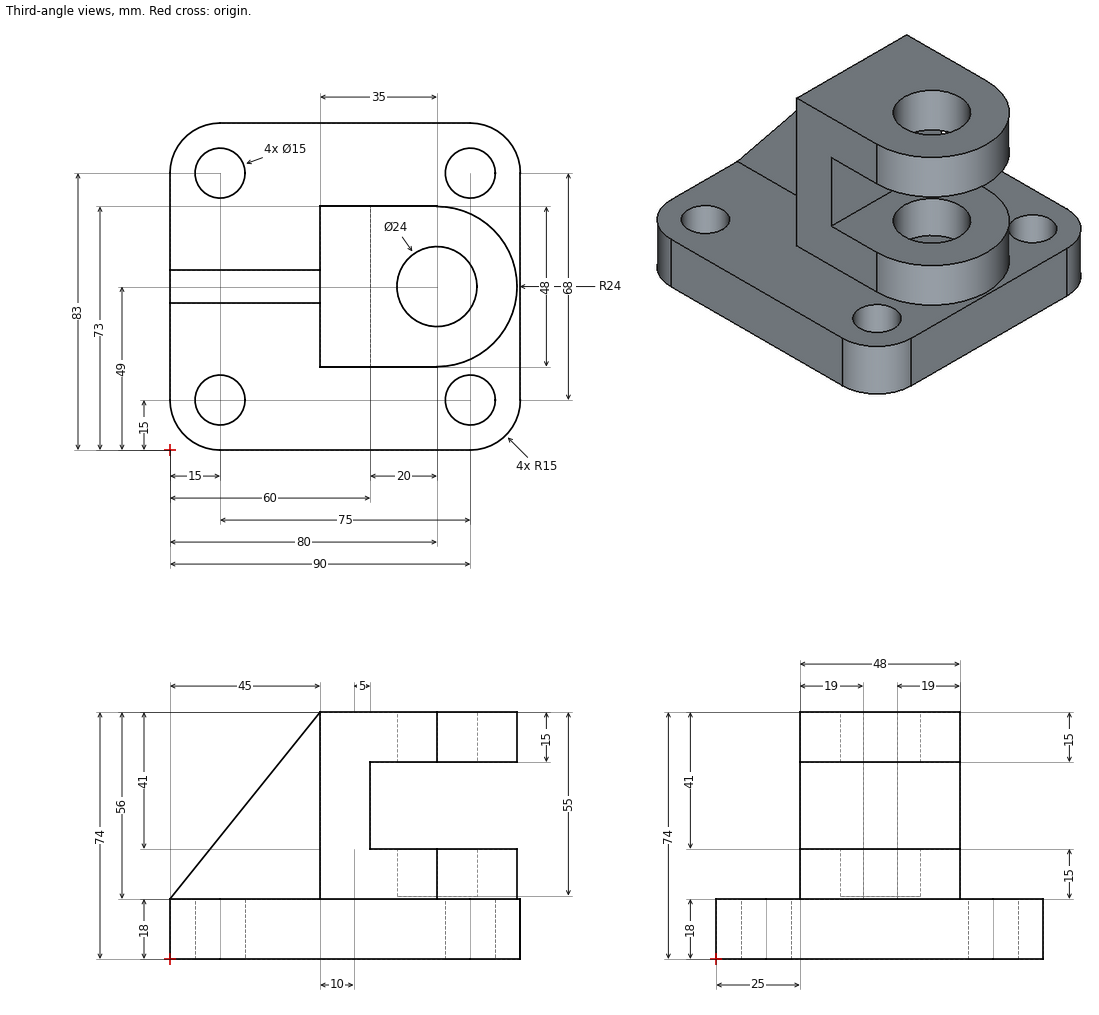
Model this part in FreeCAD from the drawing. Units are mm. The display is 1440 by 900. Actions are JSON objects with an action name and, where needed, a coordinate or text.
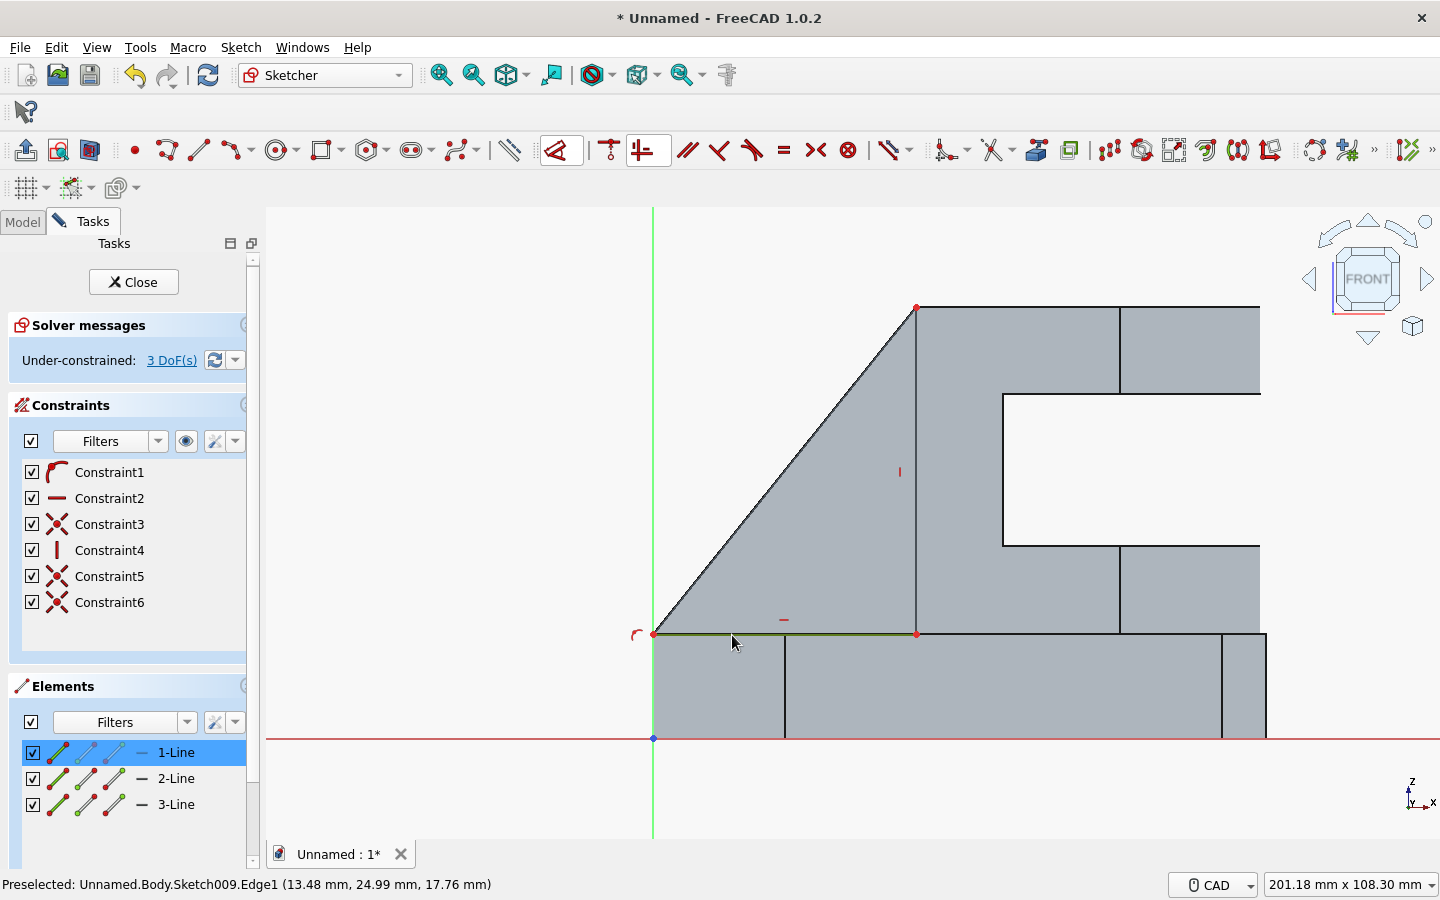
{"action": "left_click", "coordinate": [578, 150]}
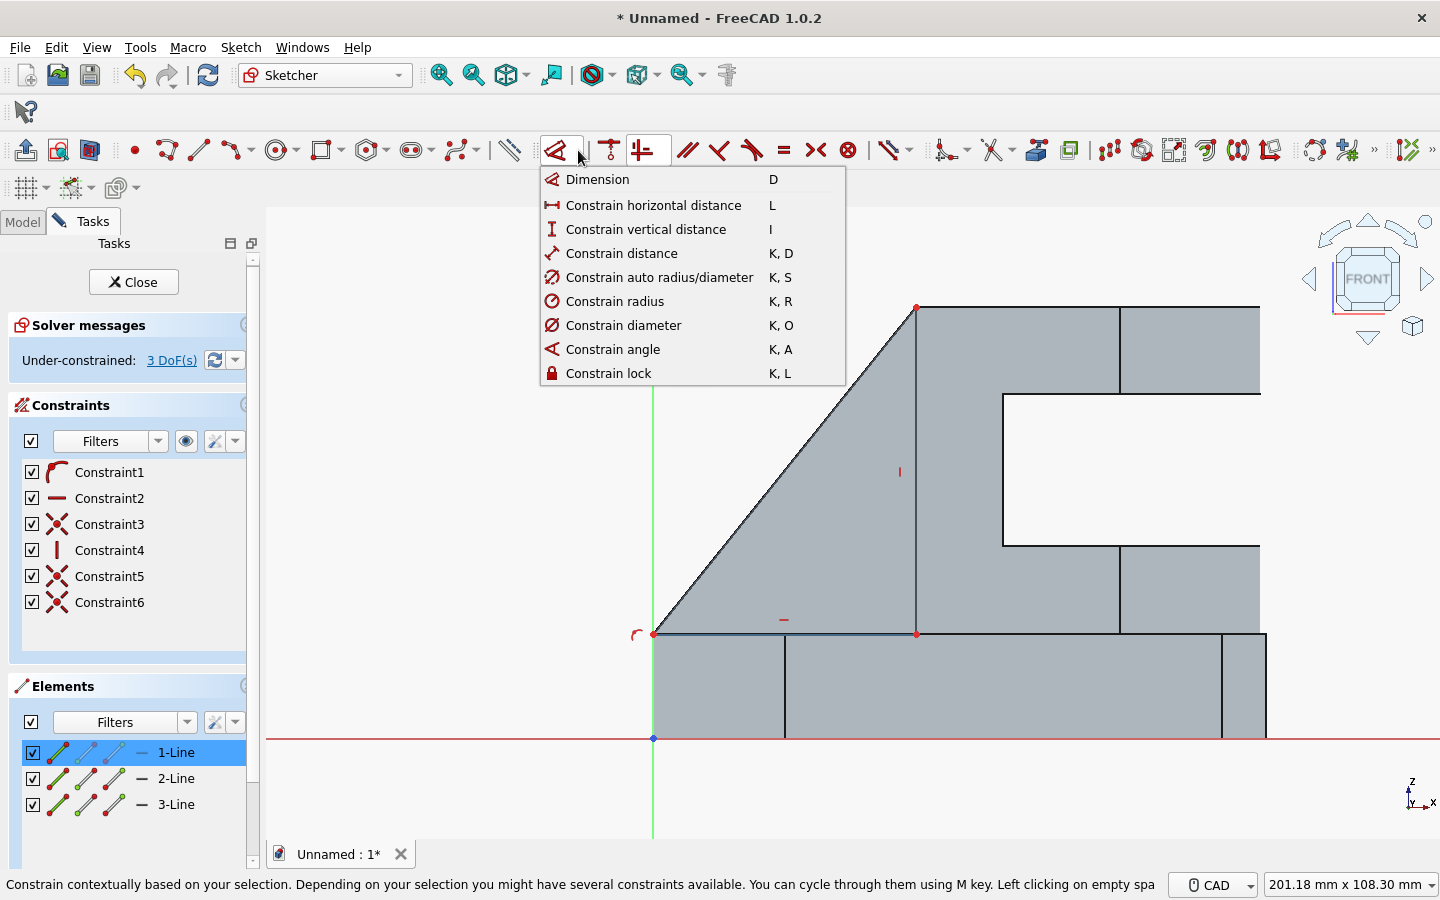
{"action": "left_click", "coordinate": [693, 205]}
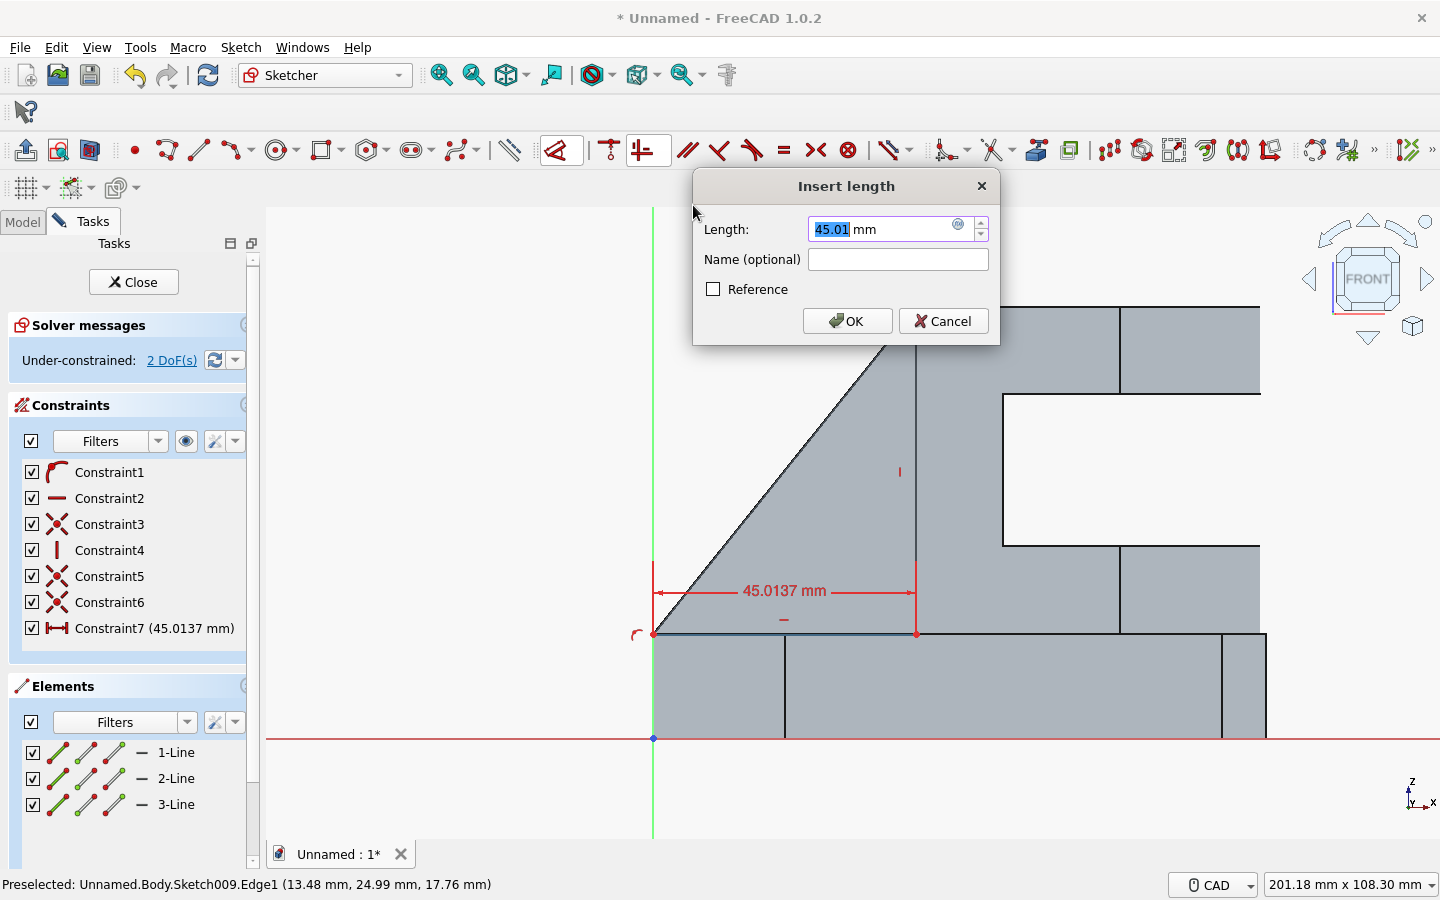
{"action": "type", "text": "45"}
{"action": "key", "text": "Return"}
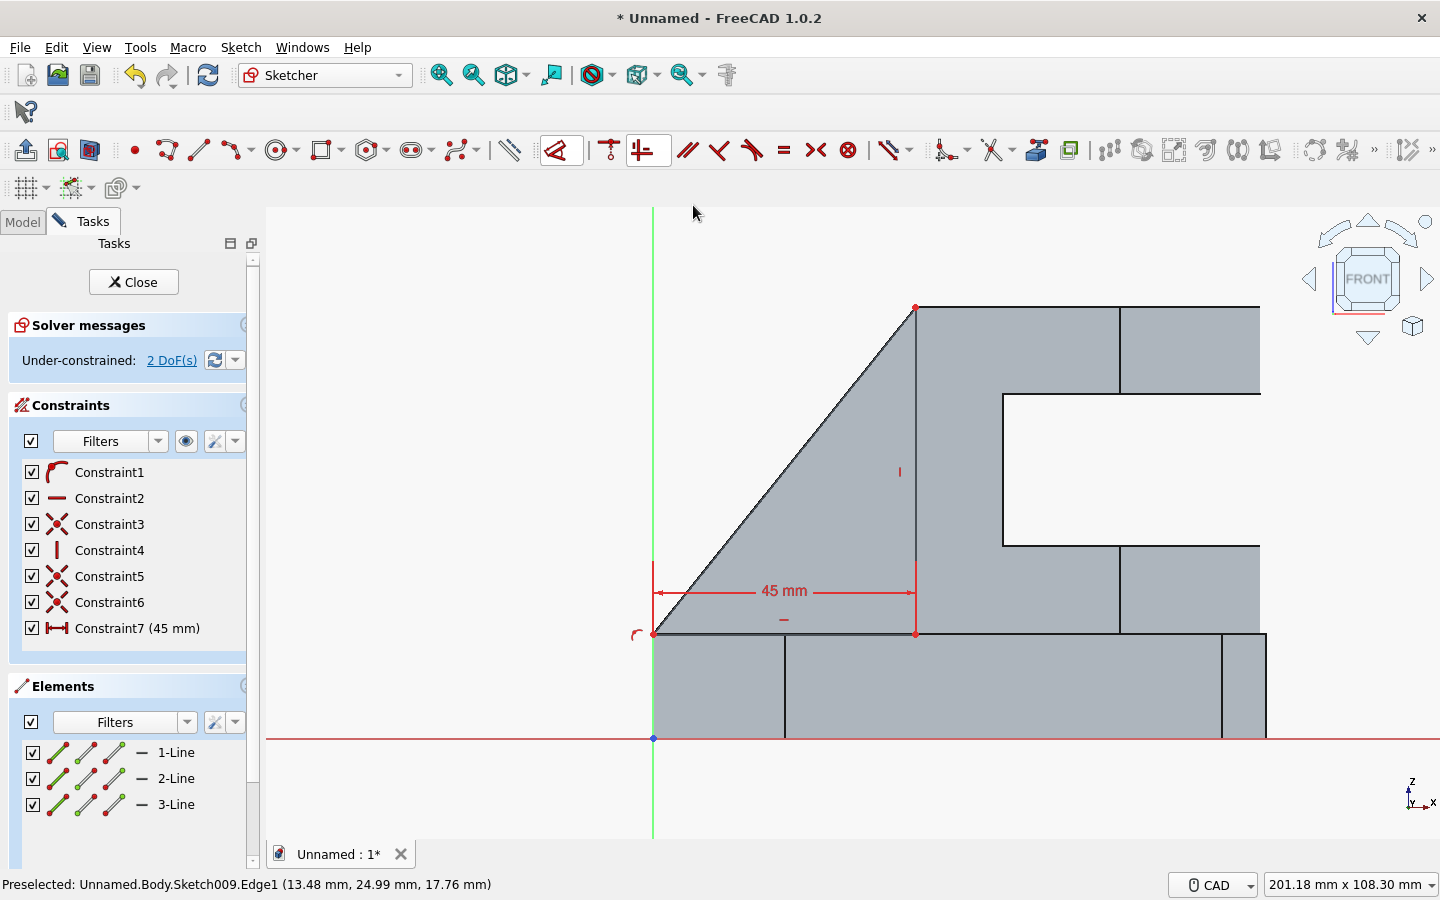
{"action": "left_click", "coordinate": [916, 537]}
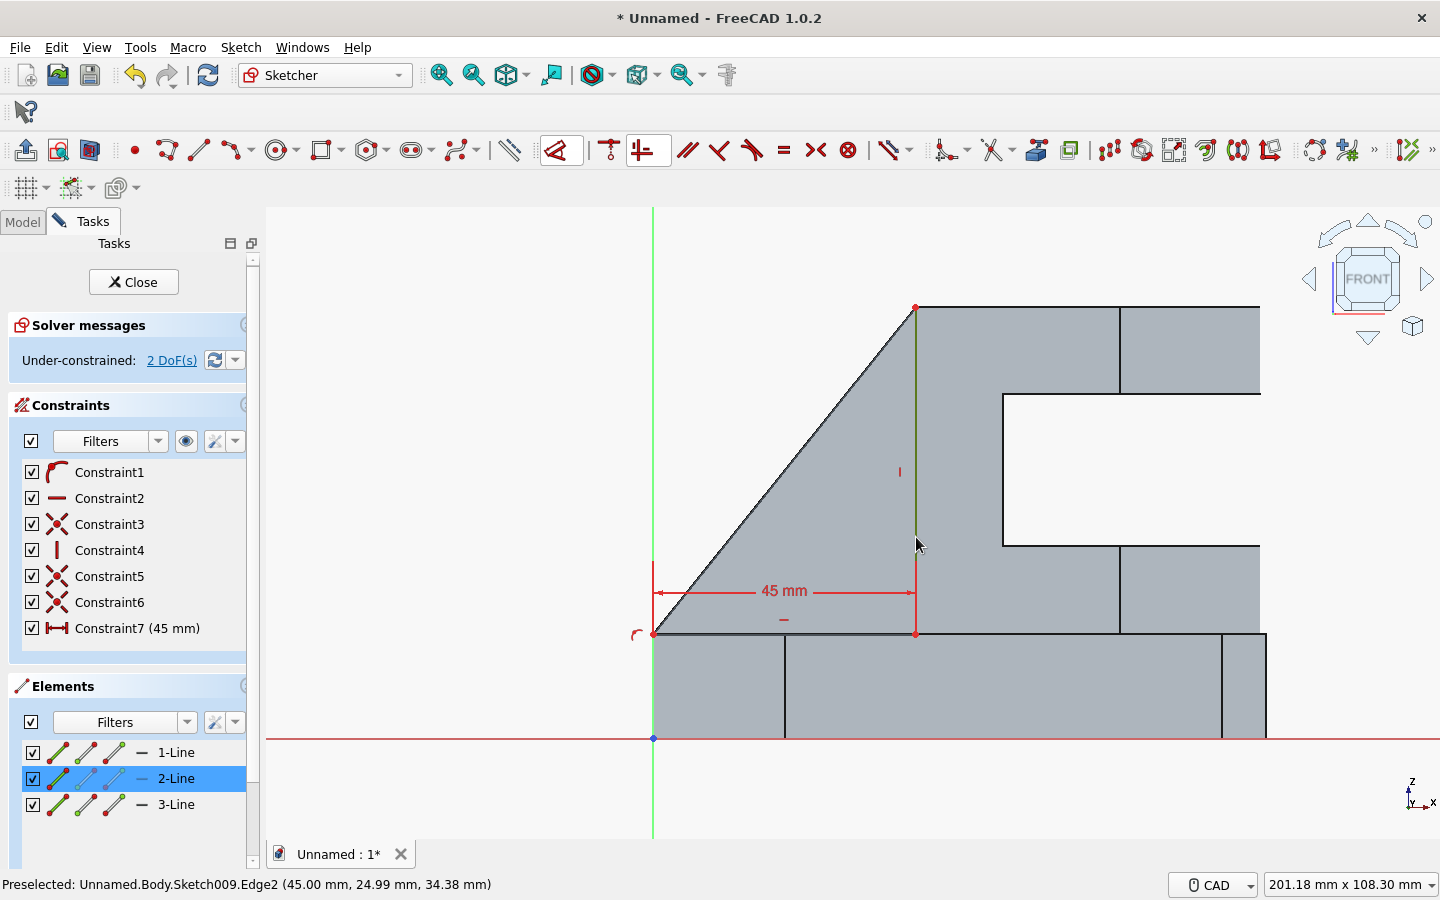
{"action": "key", "text": "i"}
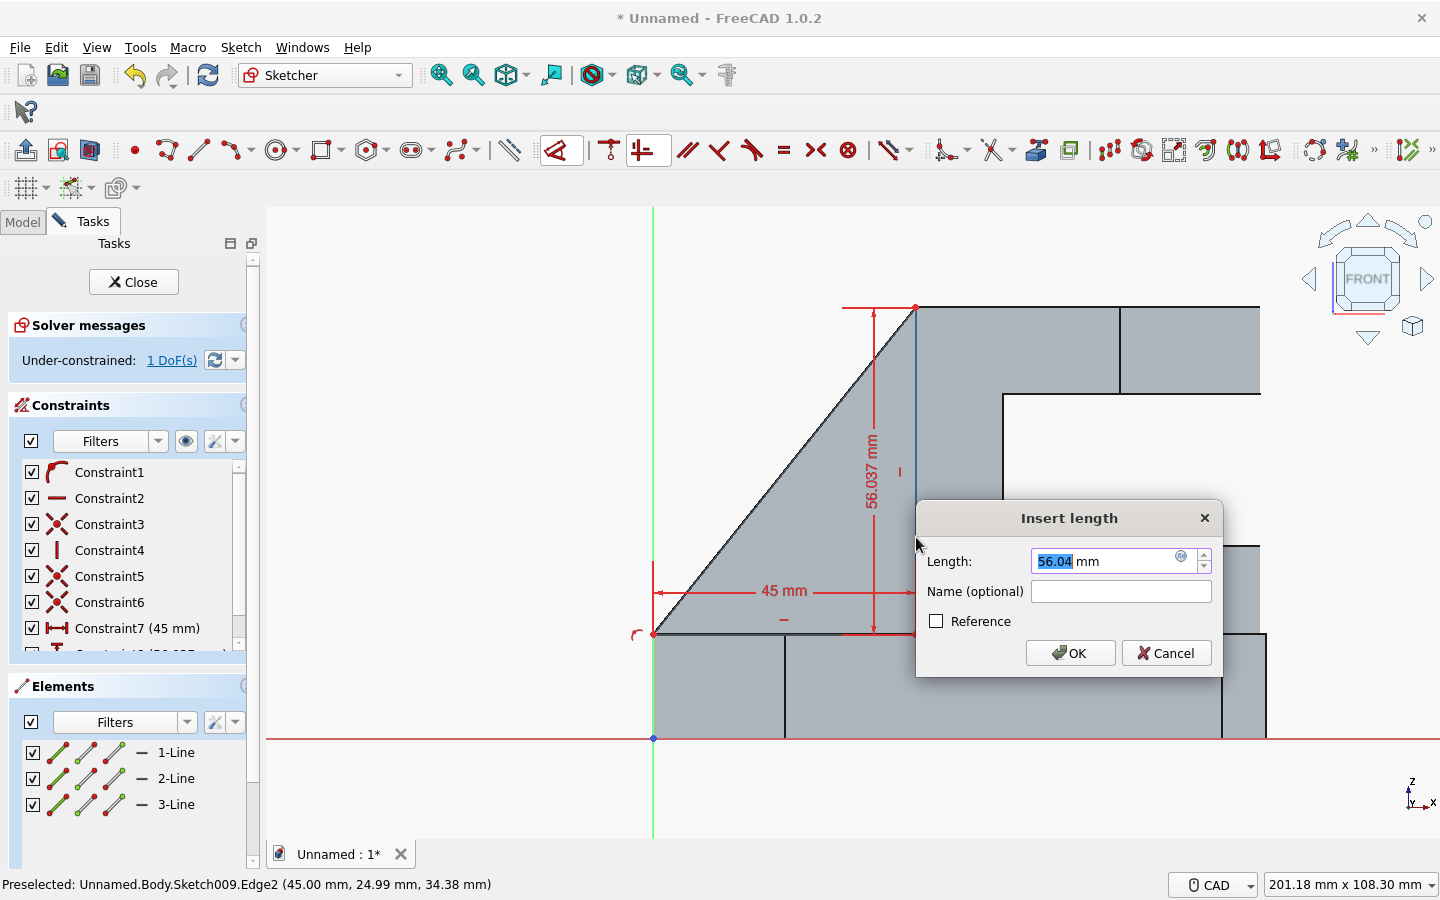
{"action": "type", "text": "56"}
{"action": "key", "text": "Return"}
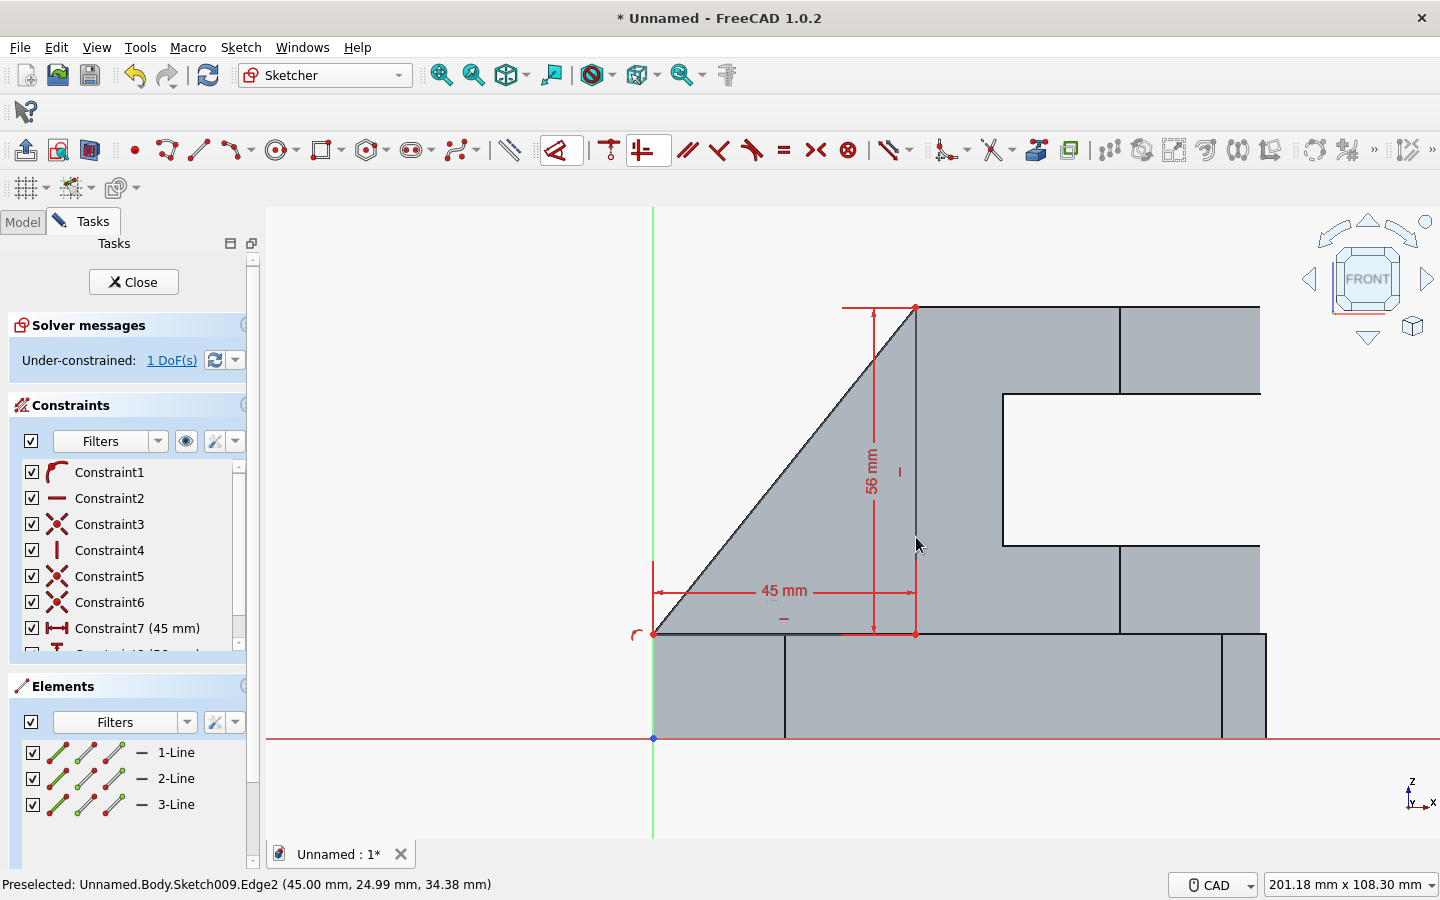
{"action": "left_click", "coordinate": [653, 635]}